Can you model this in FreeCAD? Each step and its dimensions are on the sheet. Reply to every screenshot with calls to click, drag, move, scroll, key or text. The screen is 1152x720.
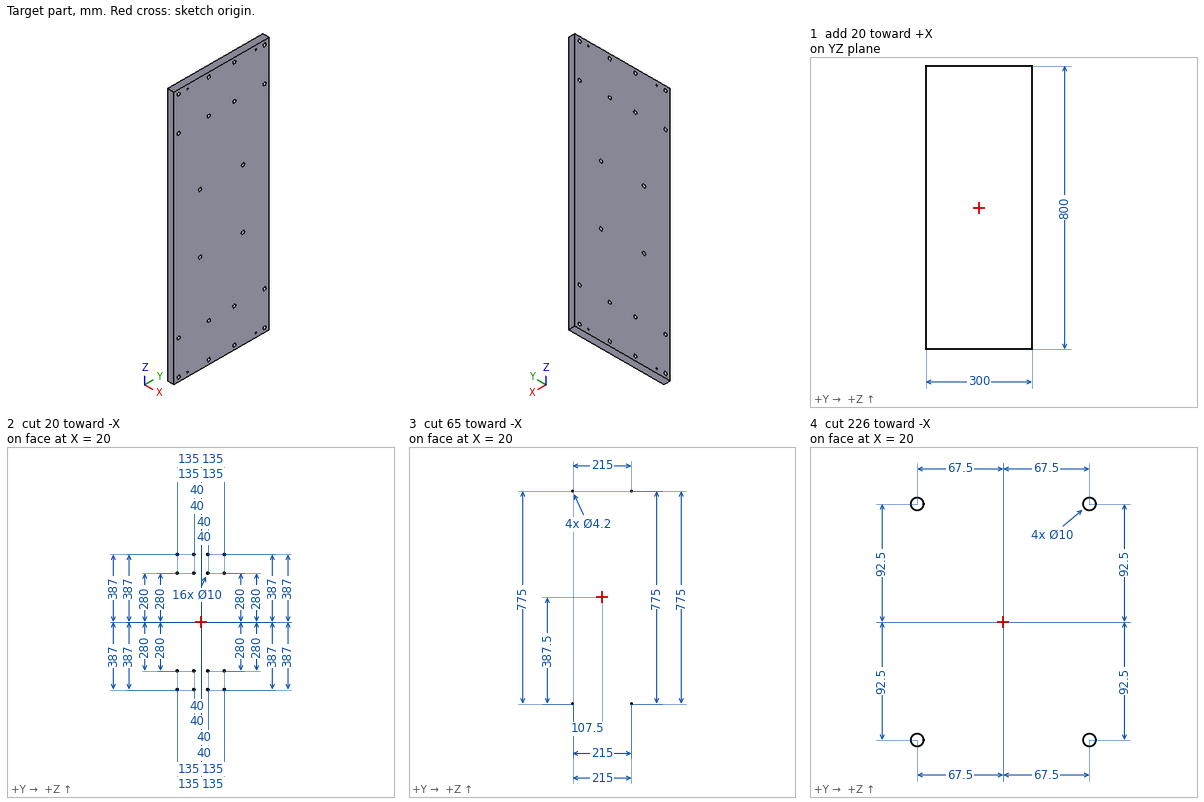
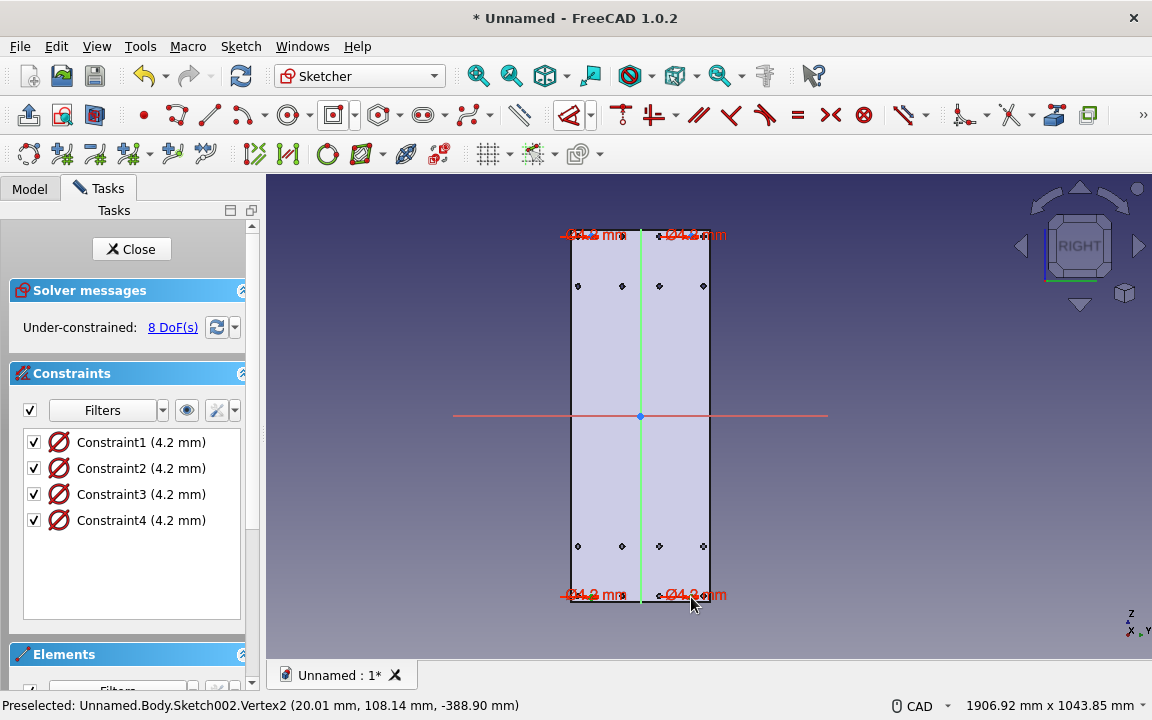
key(l)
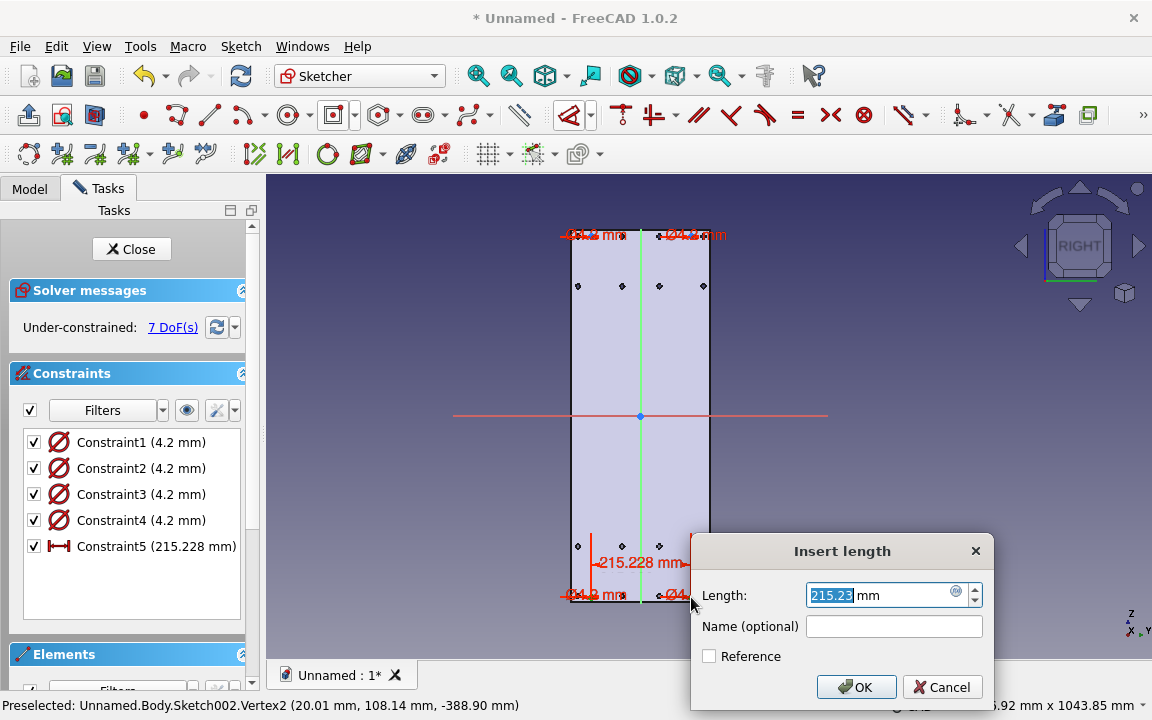
text(215)
key(Return)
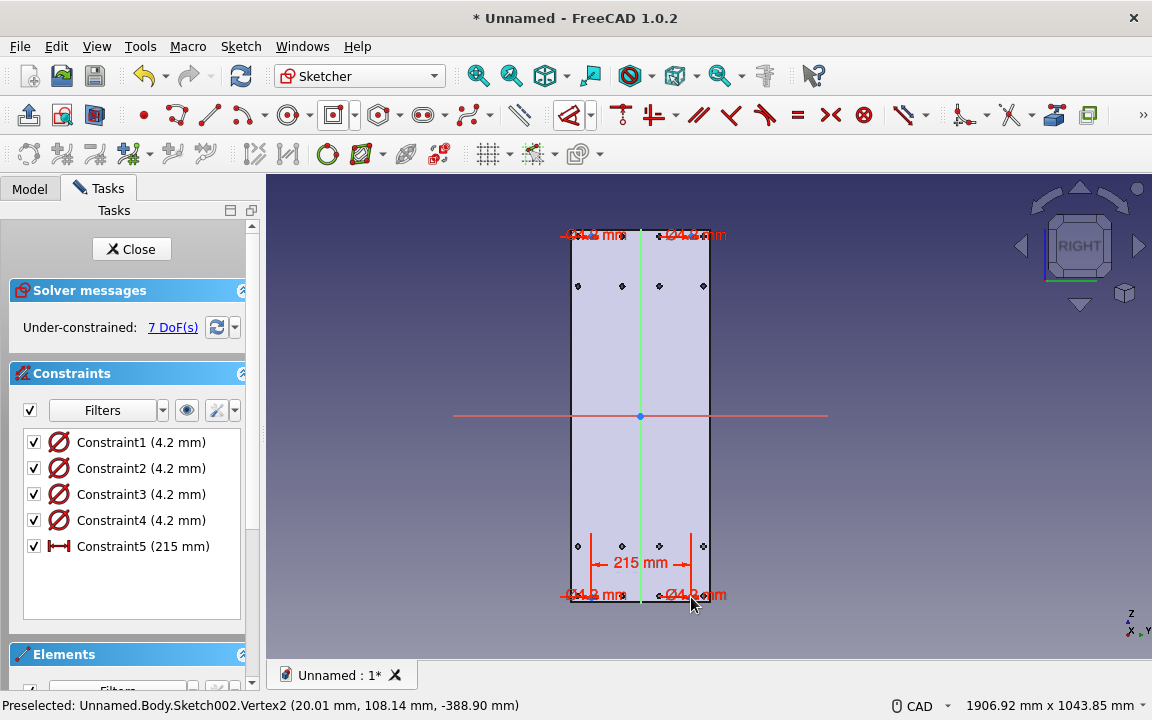
click(691, 597)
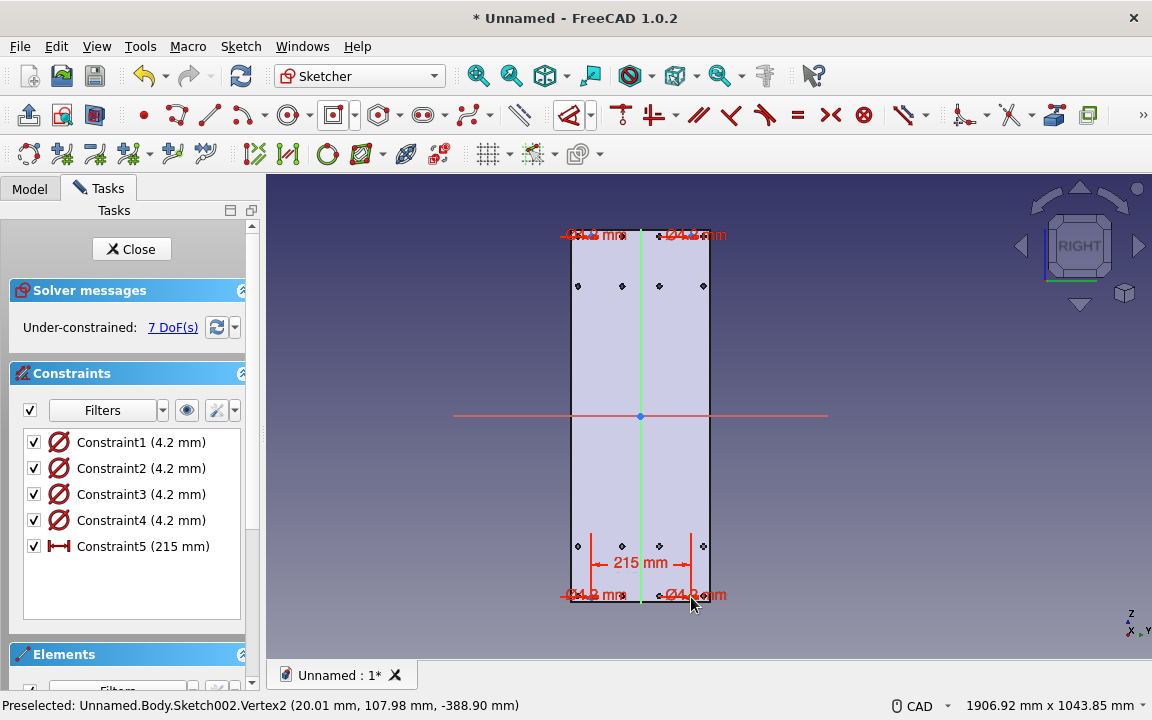
click(591, 237)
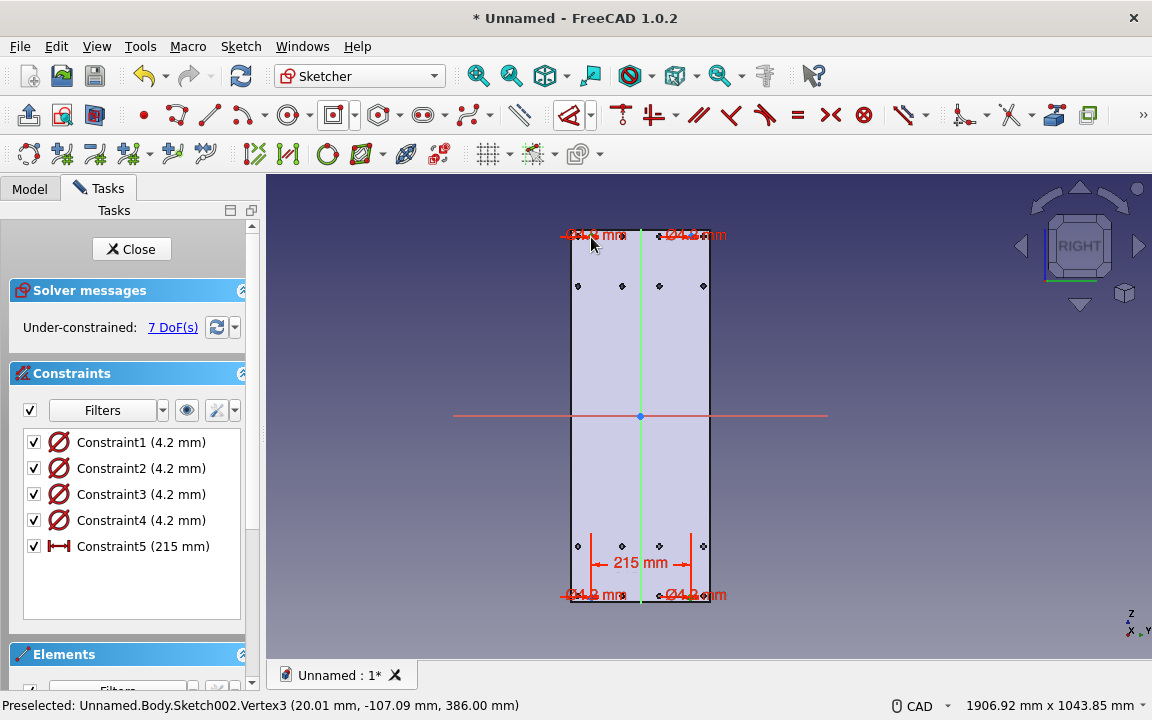
key(l)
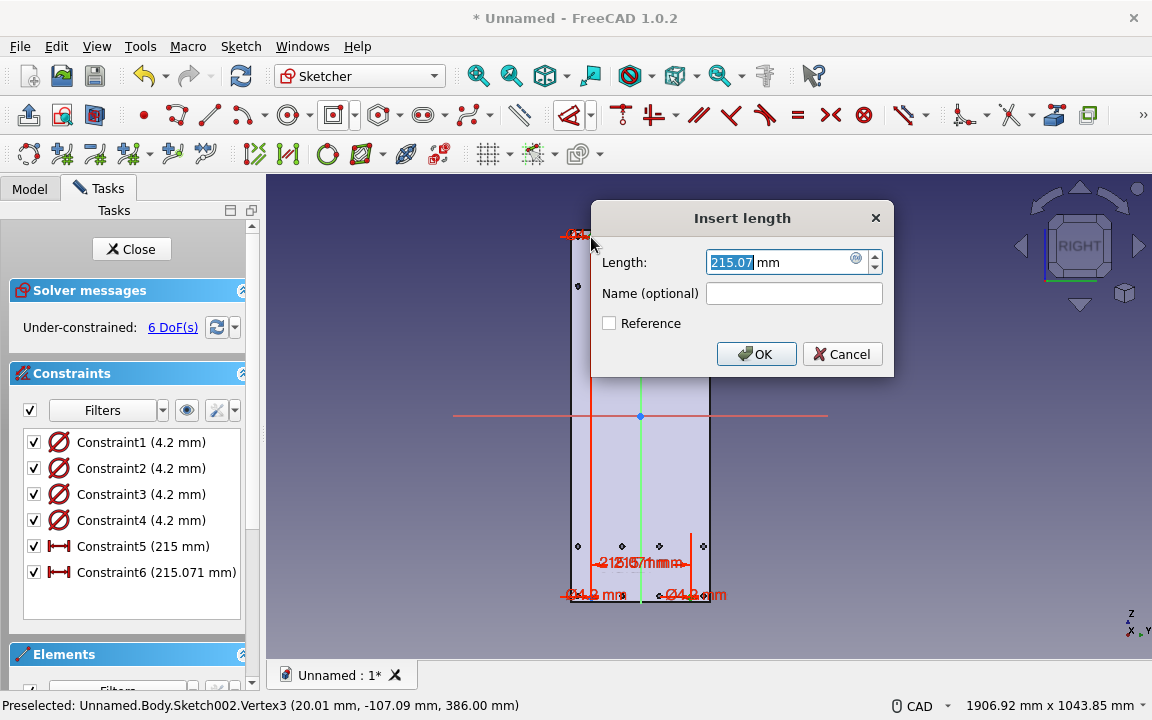
text(215)
key(Return)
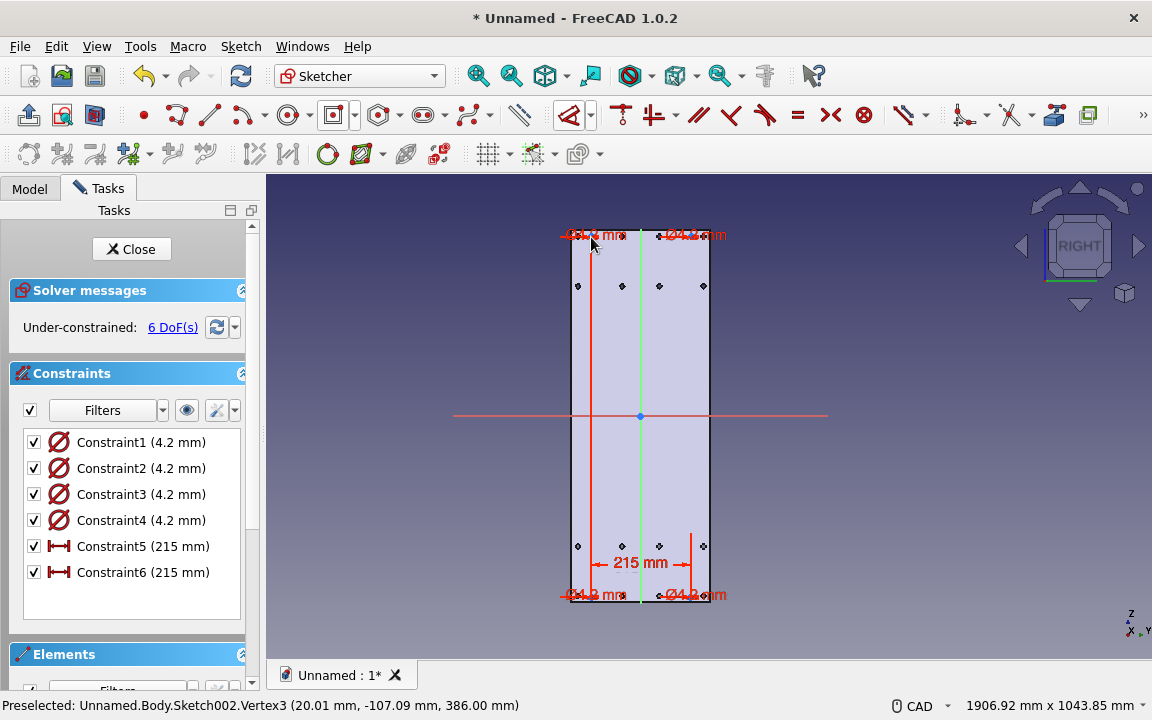
click(591, 597)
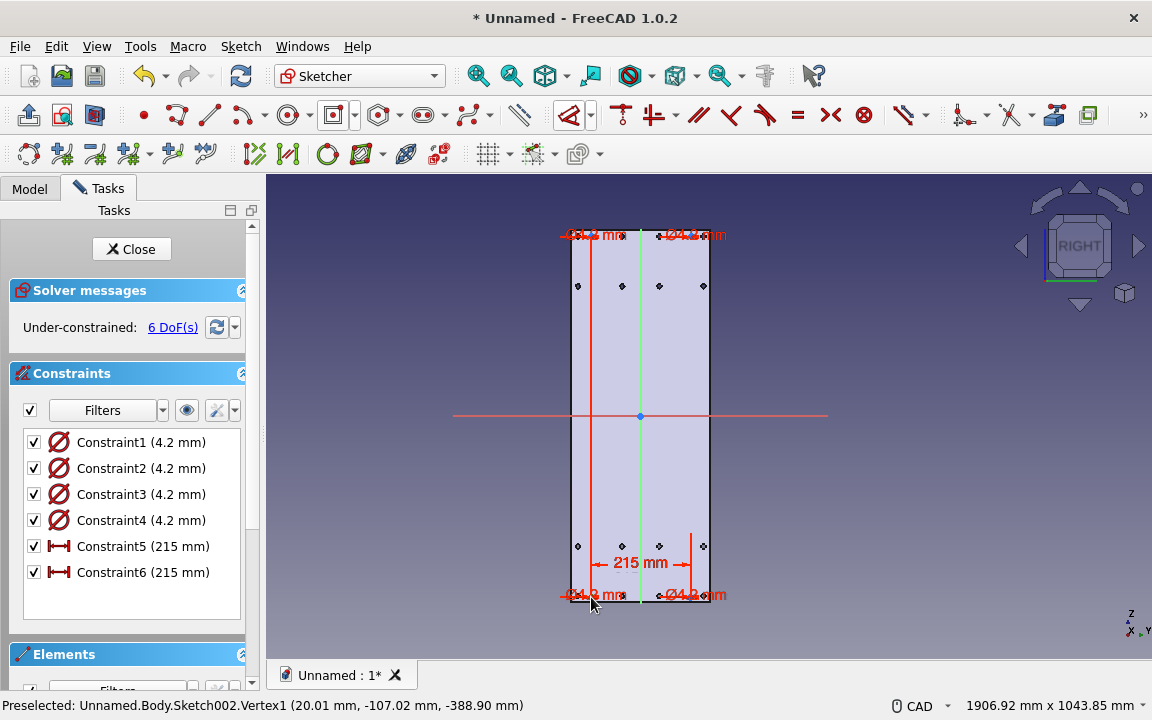
click(591, 237)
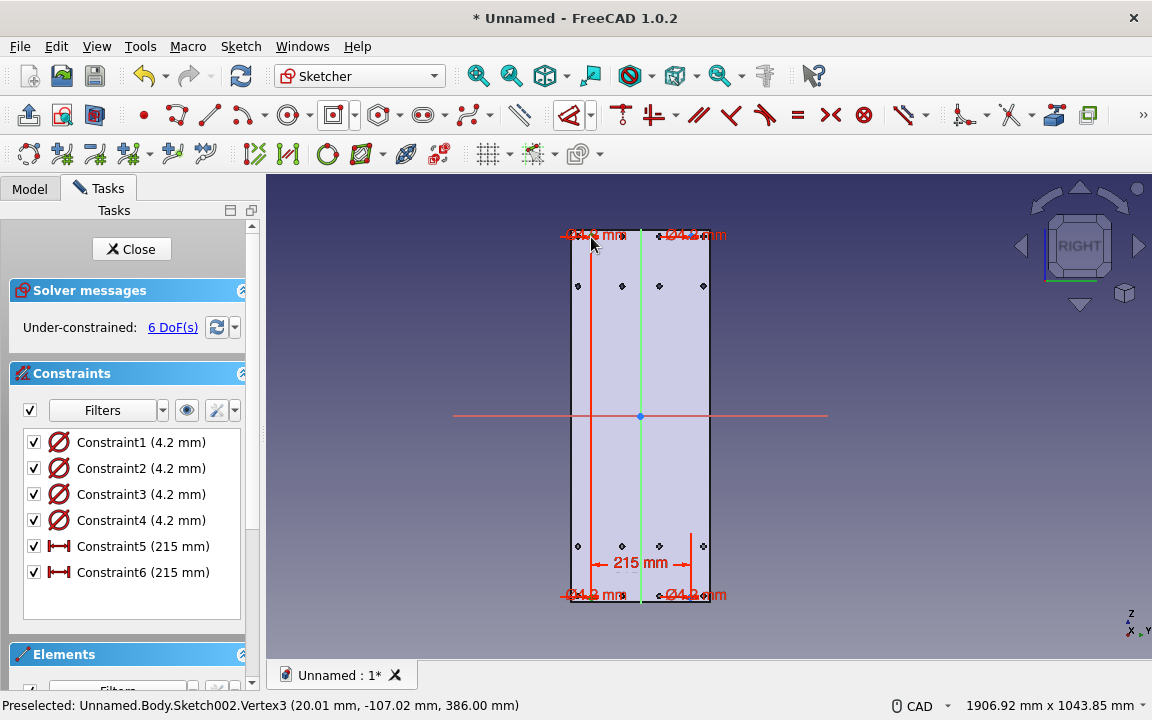
click(590, 116)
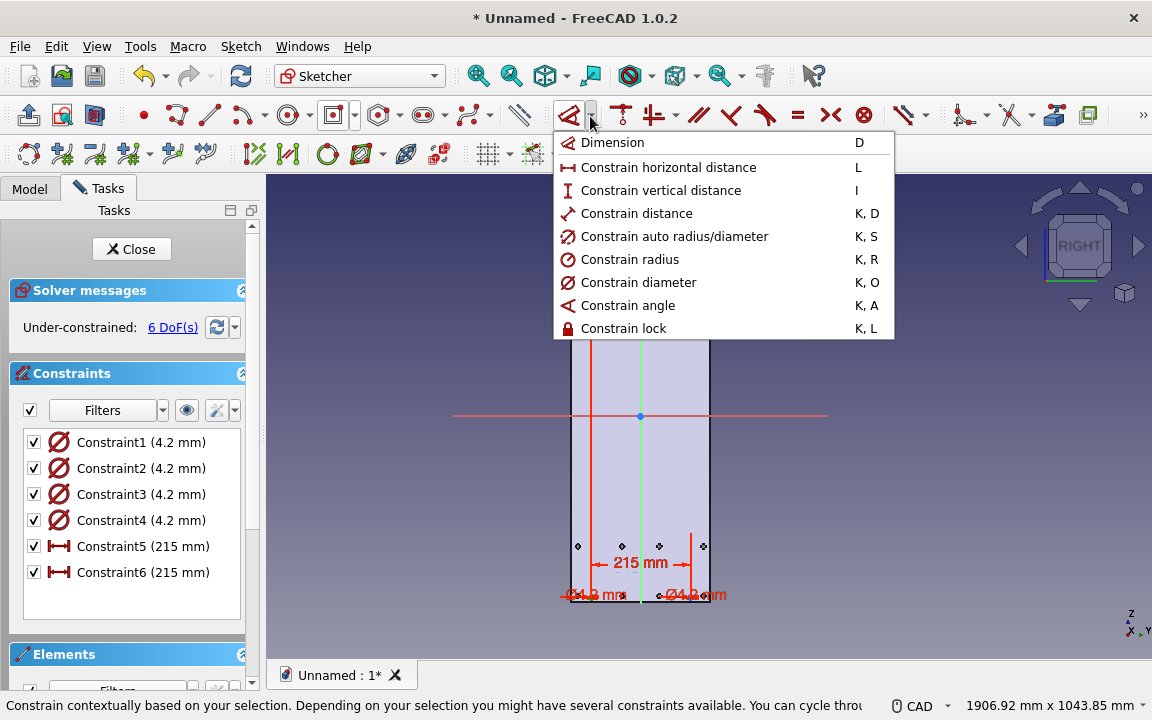
click(724, 190)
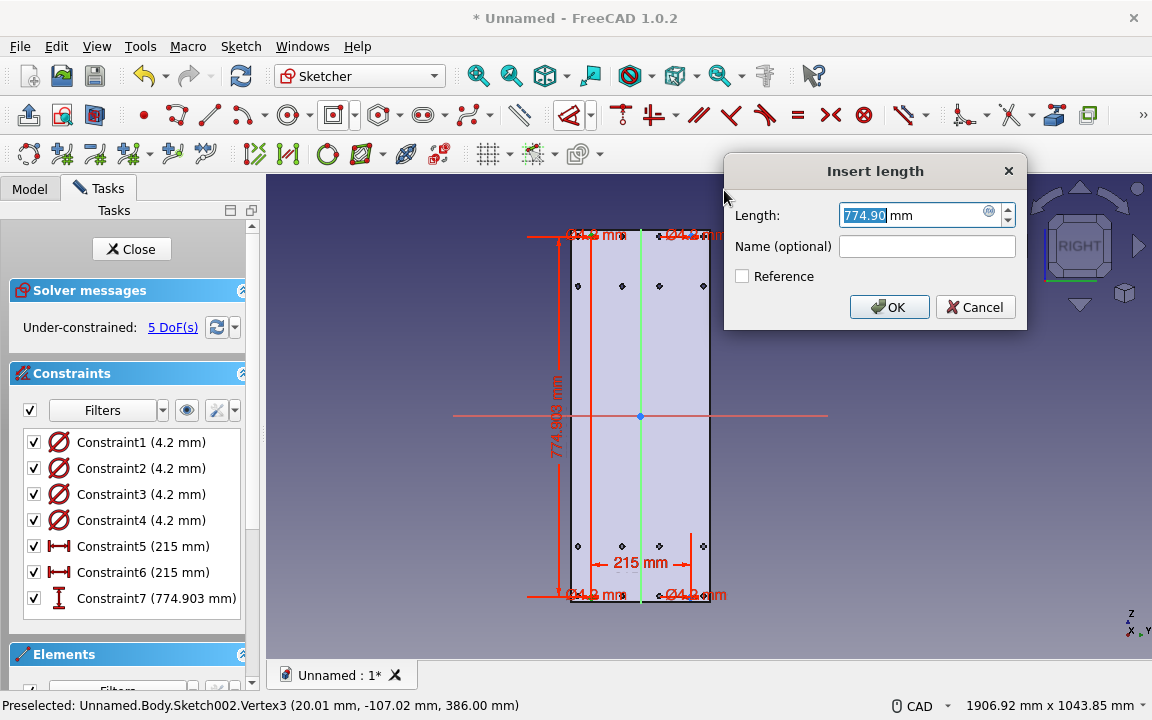
text(775)
key(Return)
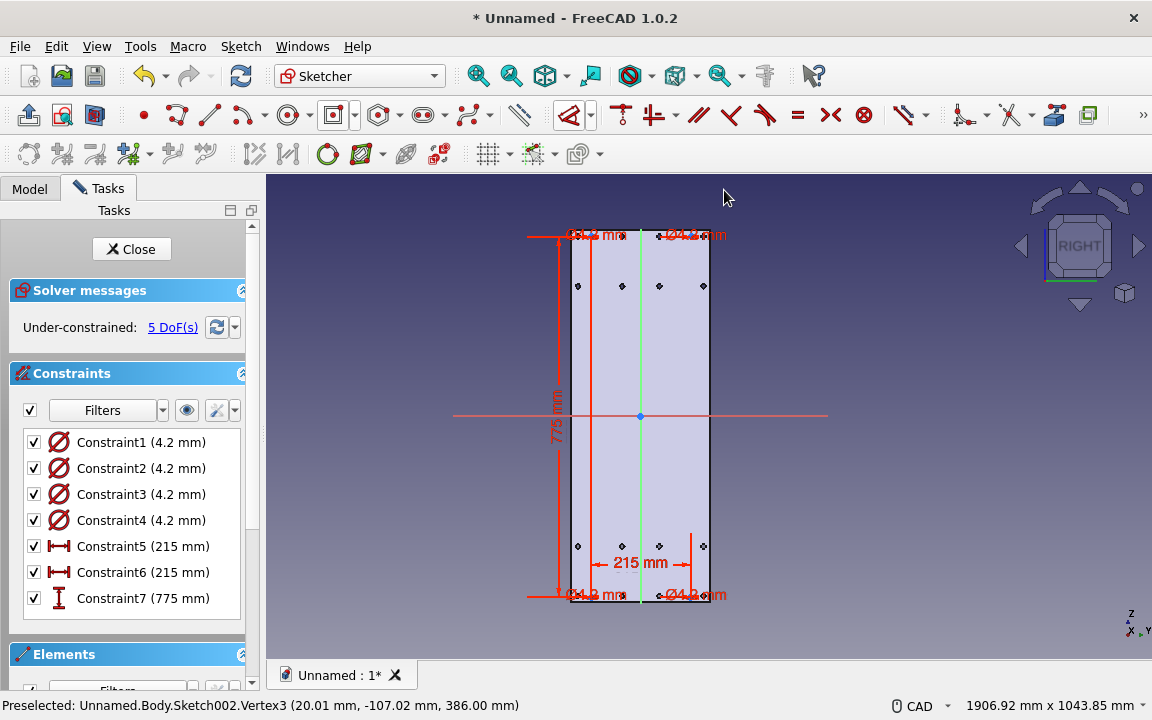
click(691, 597)